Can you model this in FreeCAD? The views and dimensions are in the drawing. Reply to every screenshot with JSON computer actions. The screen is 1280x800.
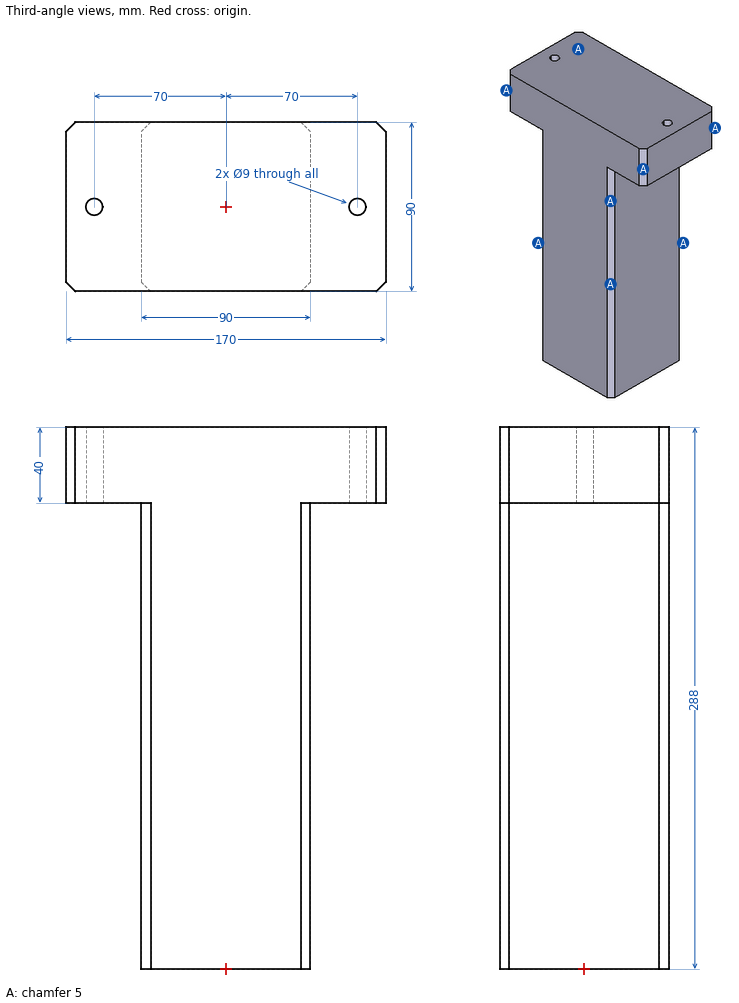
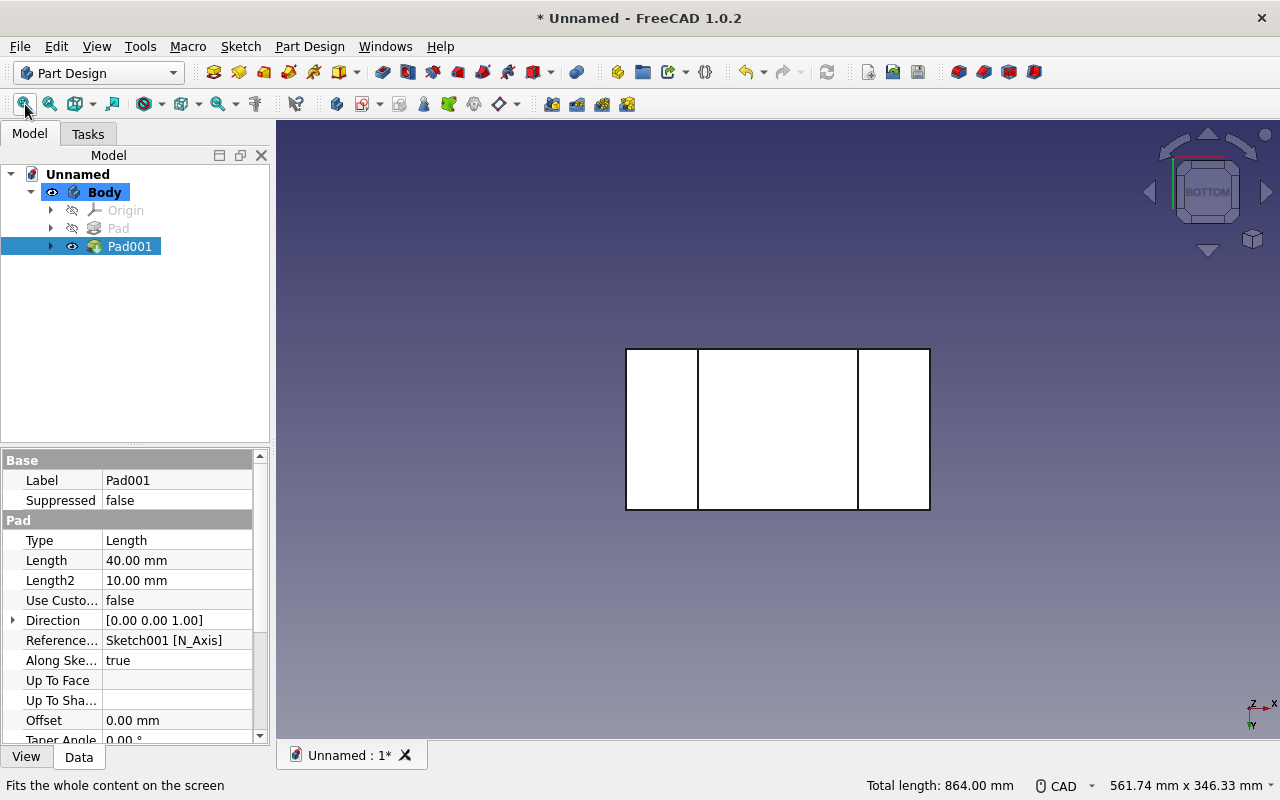
{"action": "key", "text": "4"}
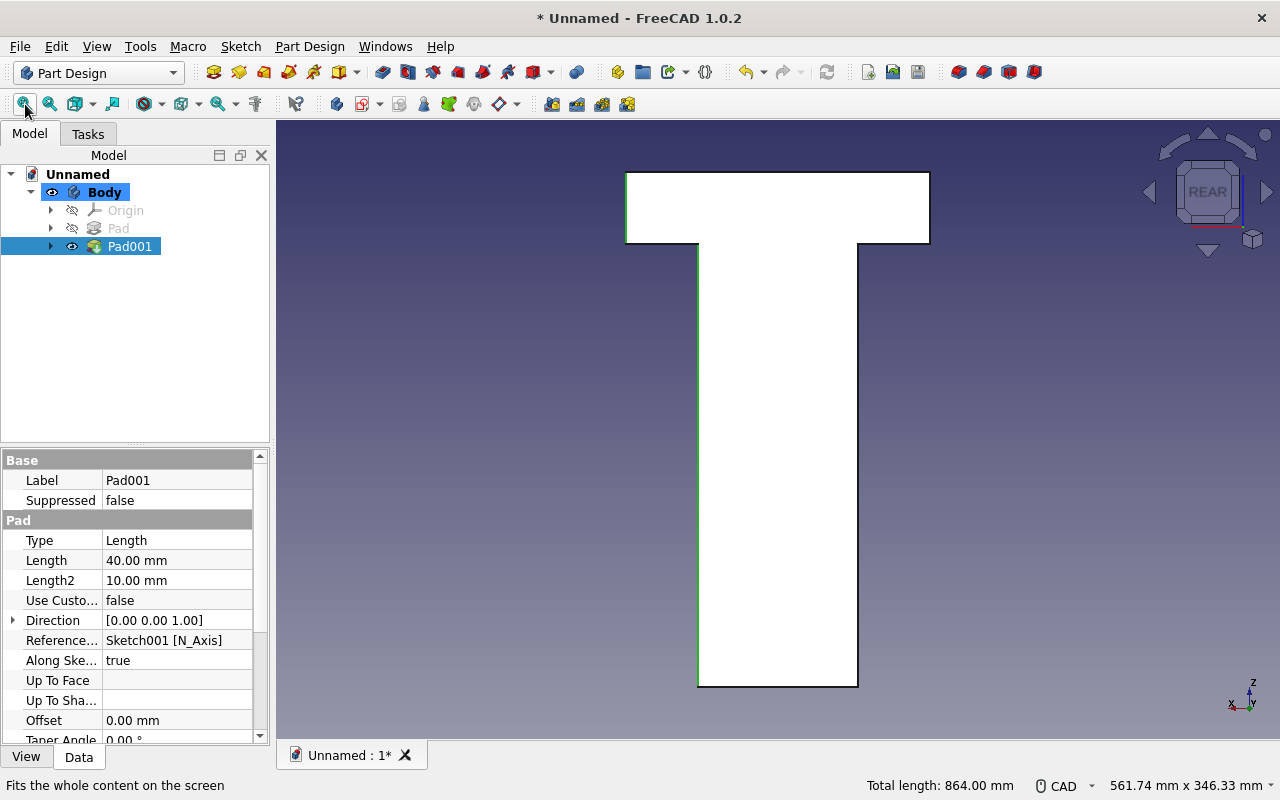
{"action": "left_click", "coordinate": [858, 464], "text": "ctrl"}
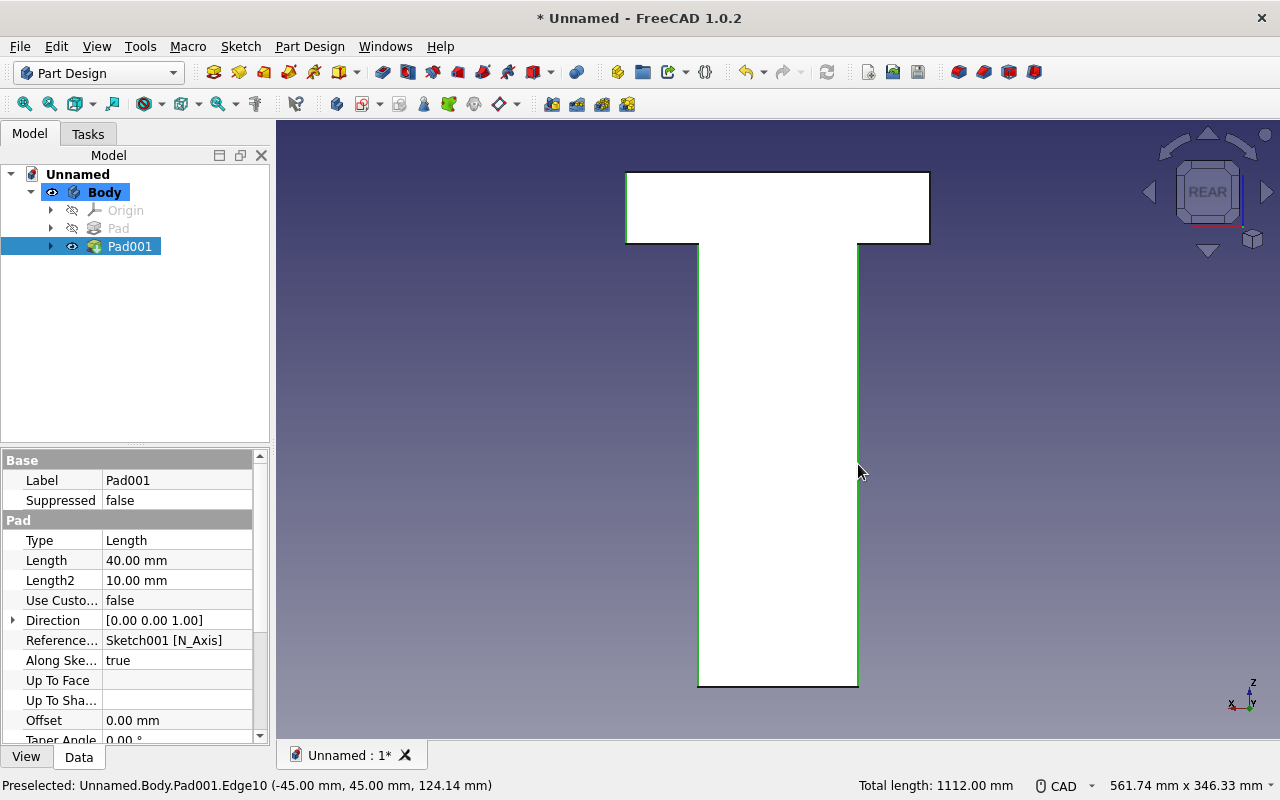
{"action": "left_click", "coordinate": [930, 207], "text": "ctrl"}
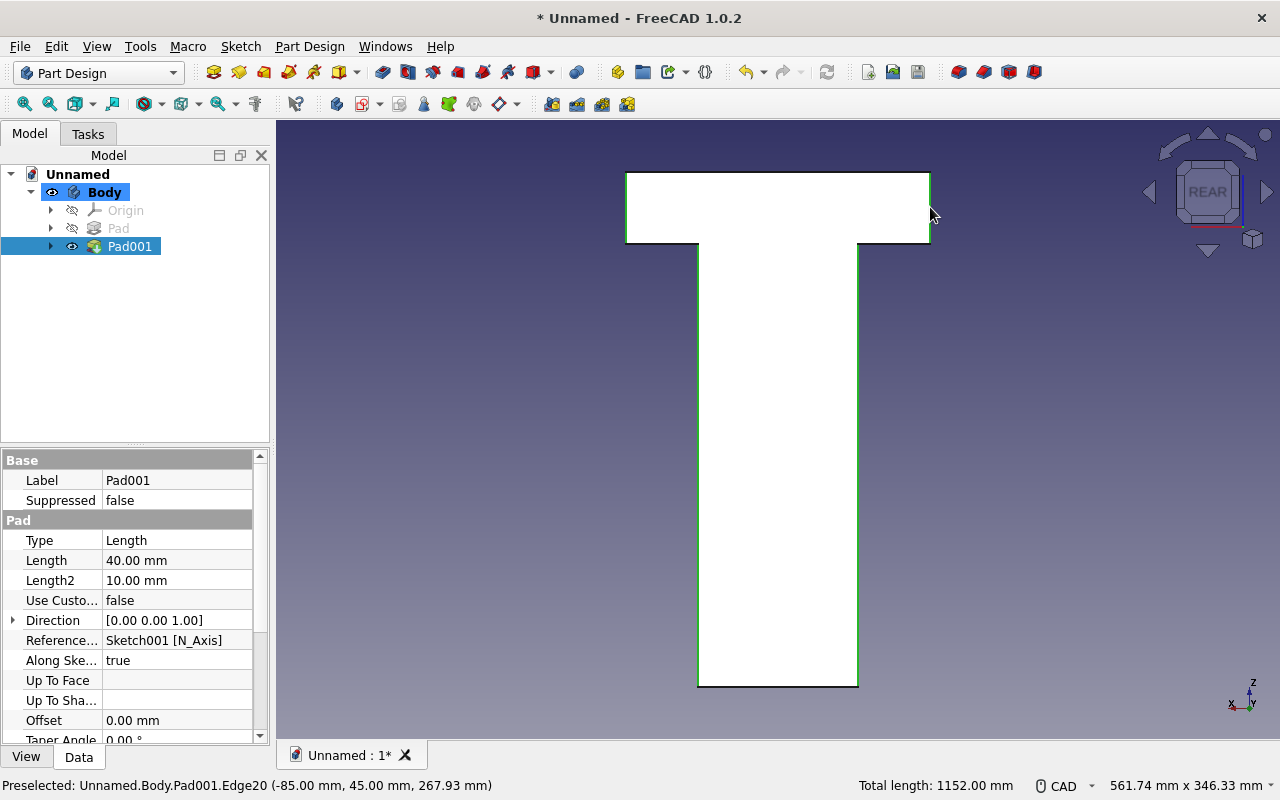
{"action": "left_click", "coordinate": [984, 72]}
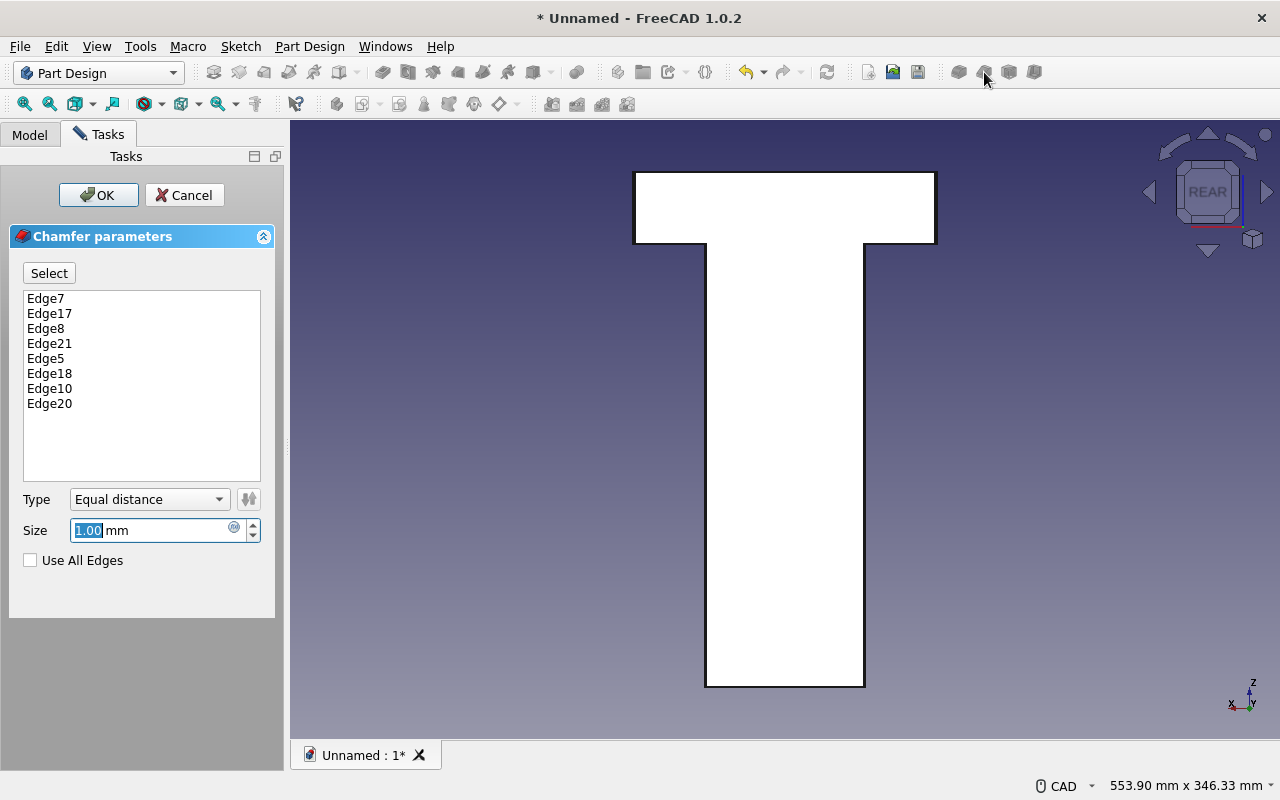
{"action": "type", "text": "5"}
{"action": "key", "text": "Tab"}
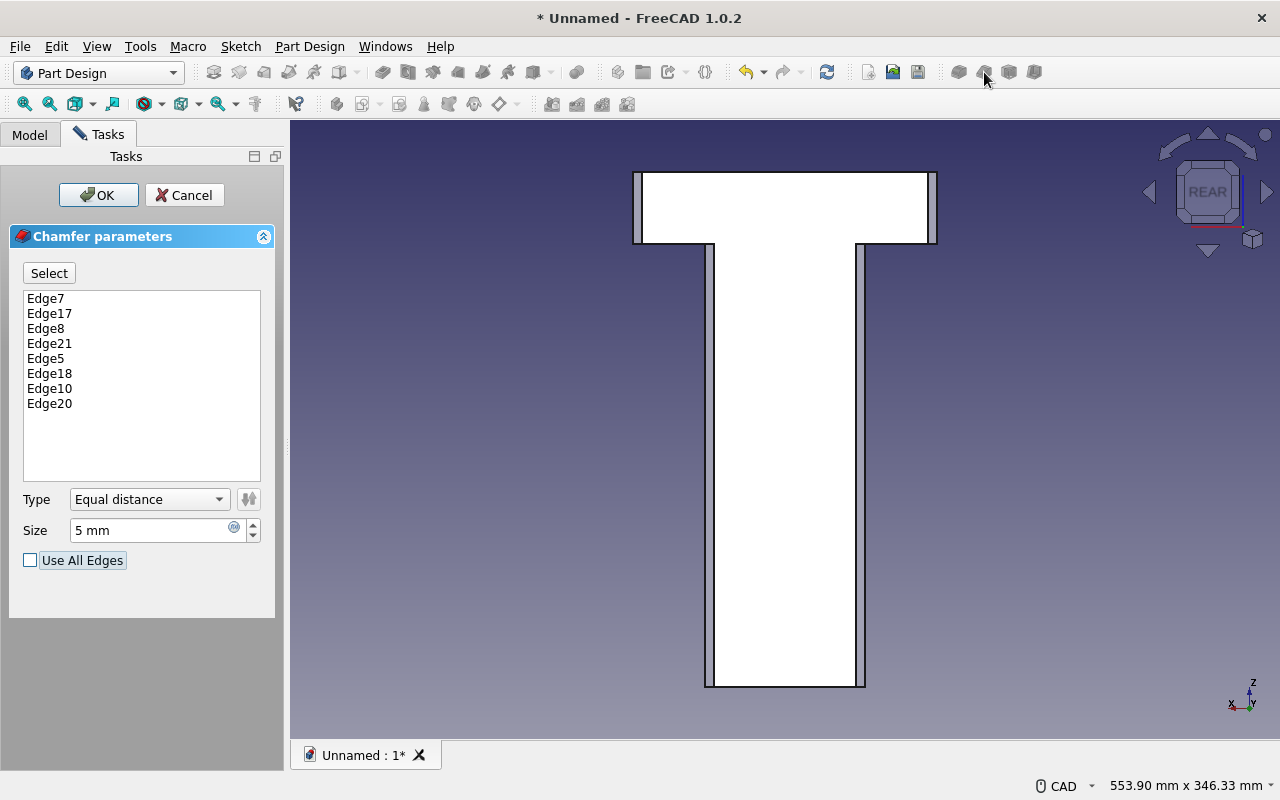
{"action": "left_click", "coordinate": [99, 195]}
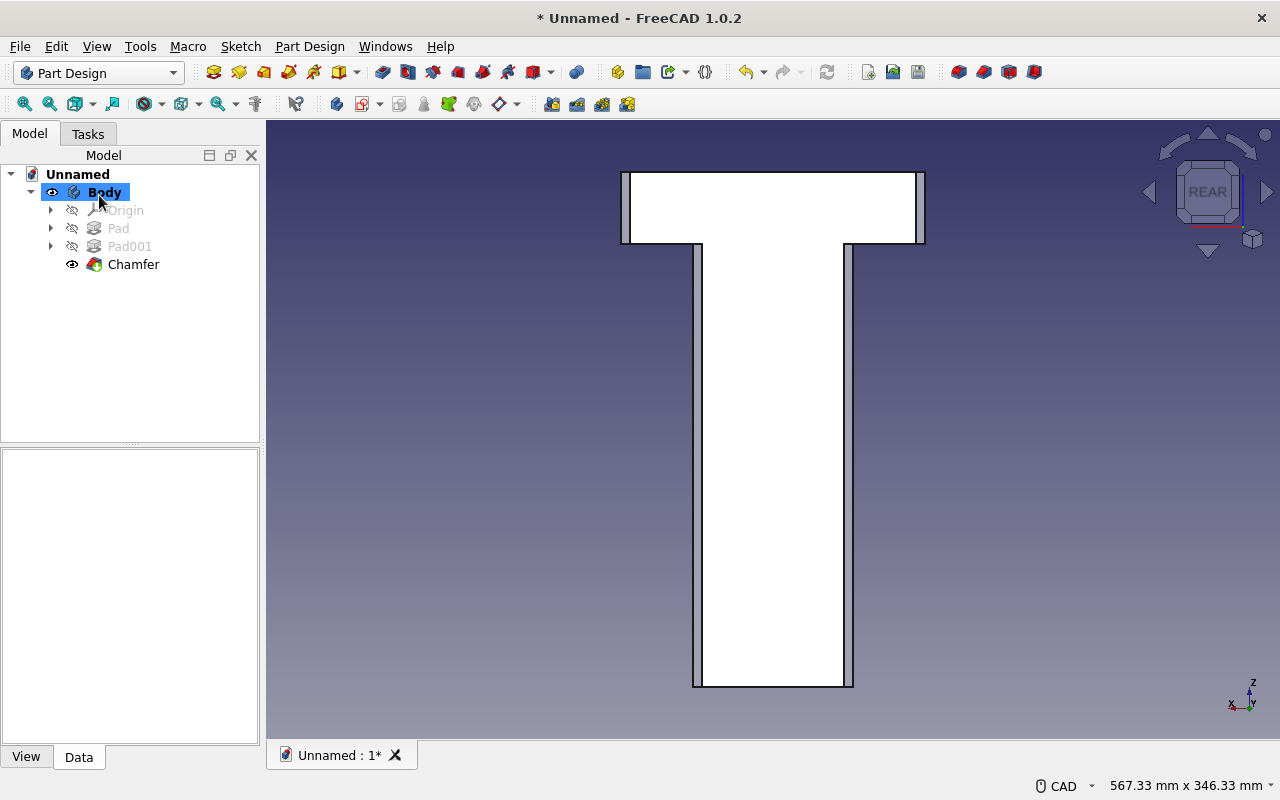
{"action": "key", "text": "5"}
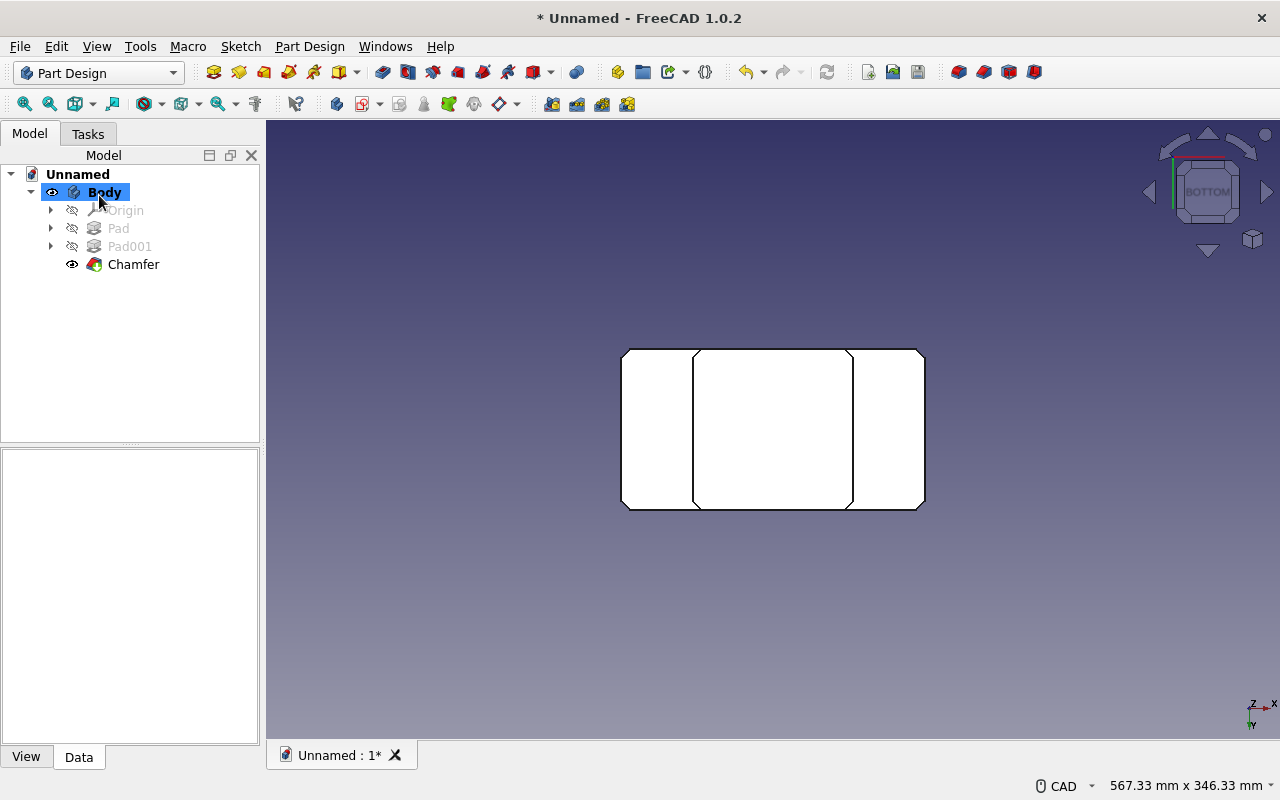
{"action": "left_click", "coordinate": [25, 104]}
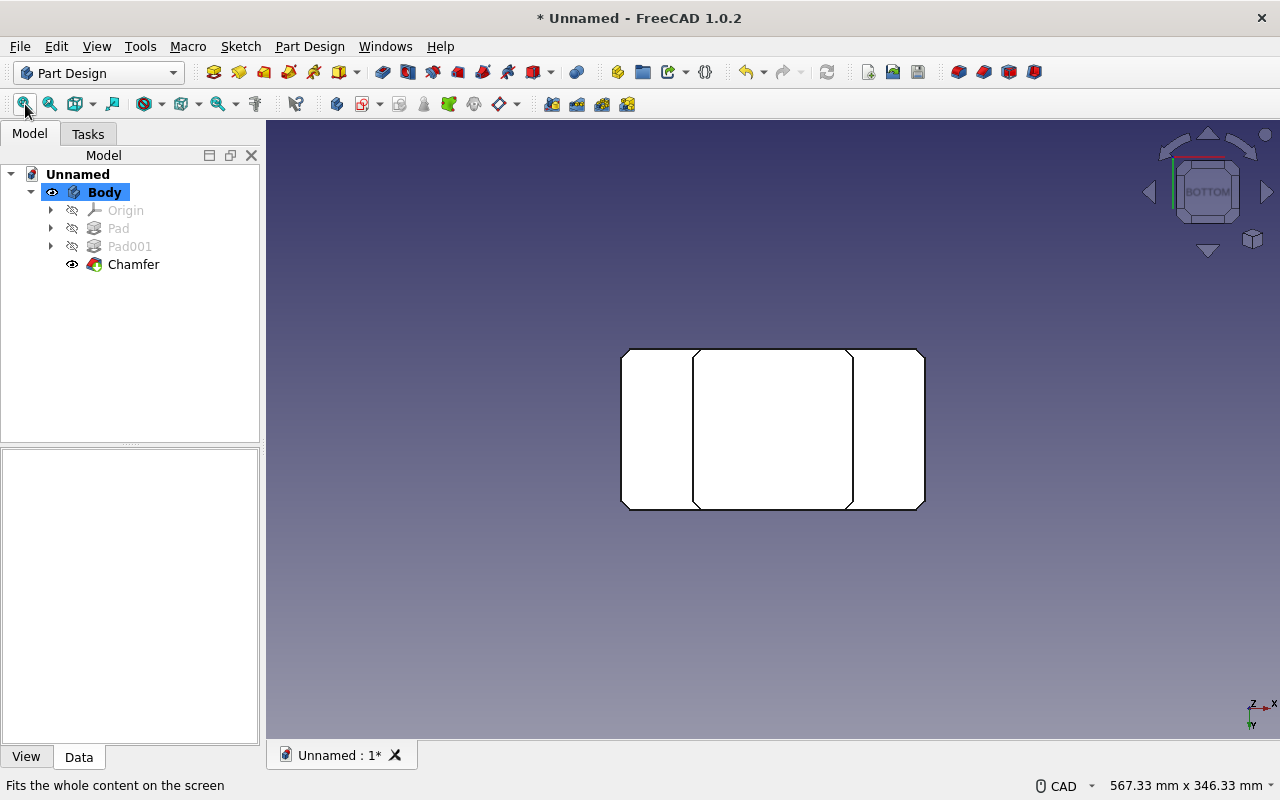
{"action": "left_click", "coordinate": [885, 474]}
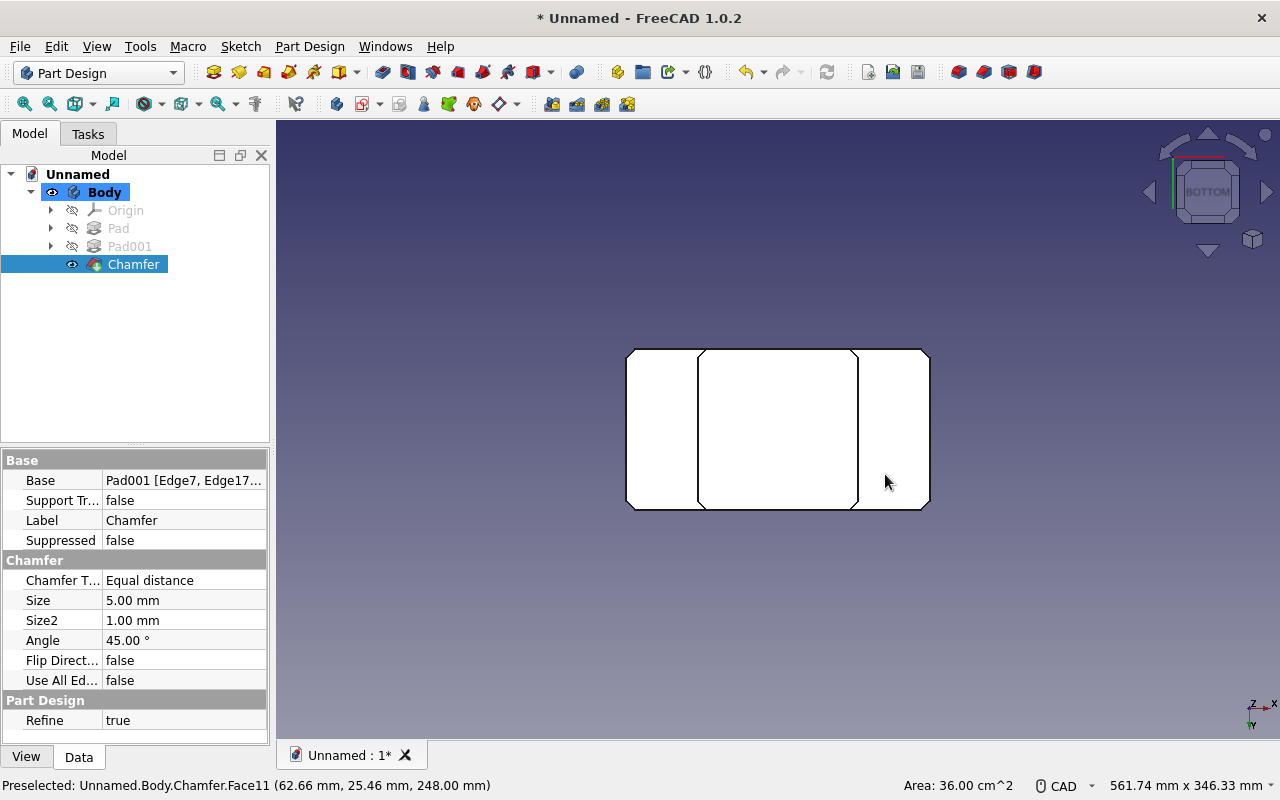
{"action": "left_click", "coordinate": [362, 104]}